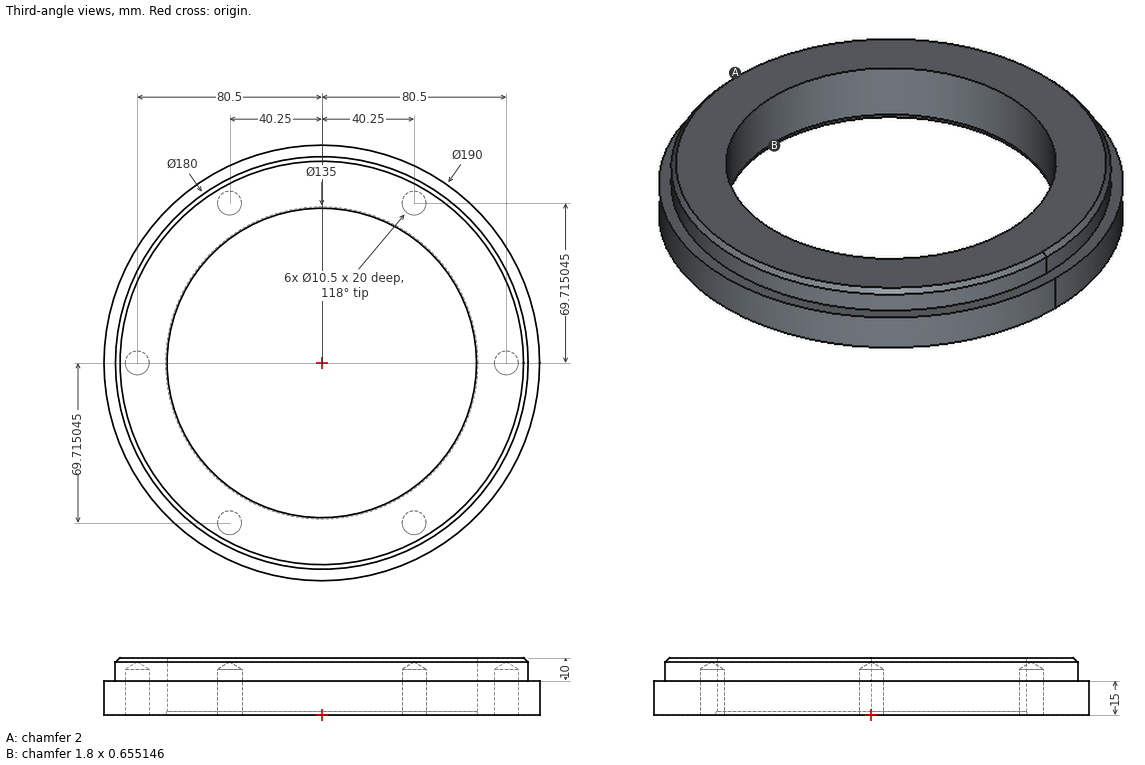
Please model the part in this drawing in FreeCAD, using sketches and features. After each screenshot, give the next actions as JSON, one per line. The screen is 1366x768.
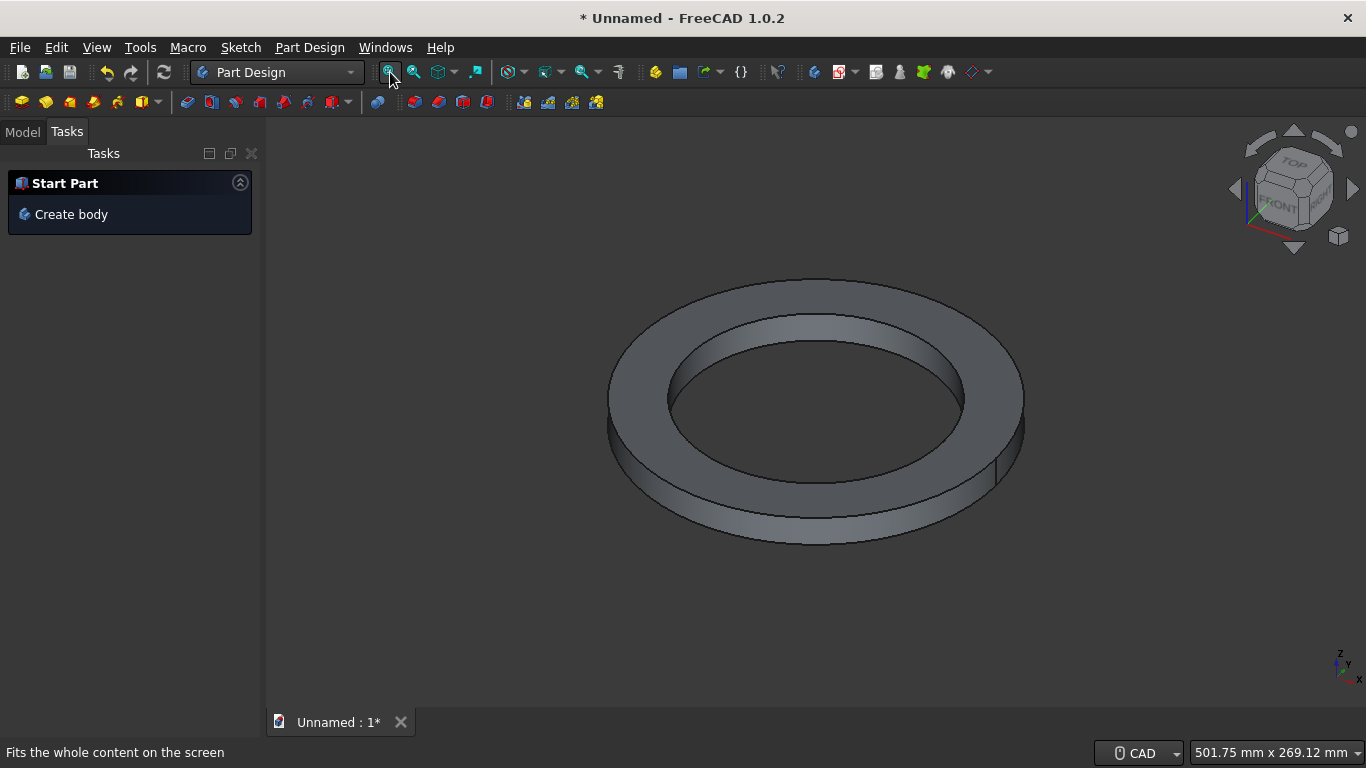
{"action": "left_click", "coordinate": [971, 449]}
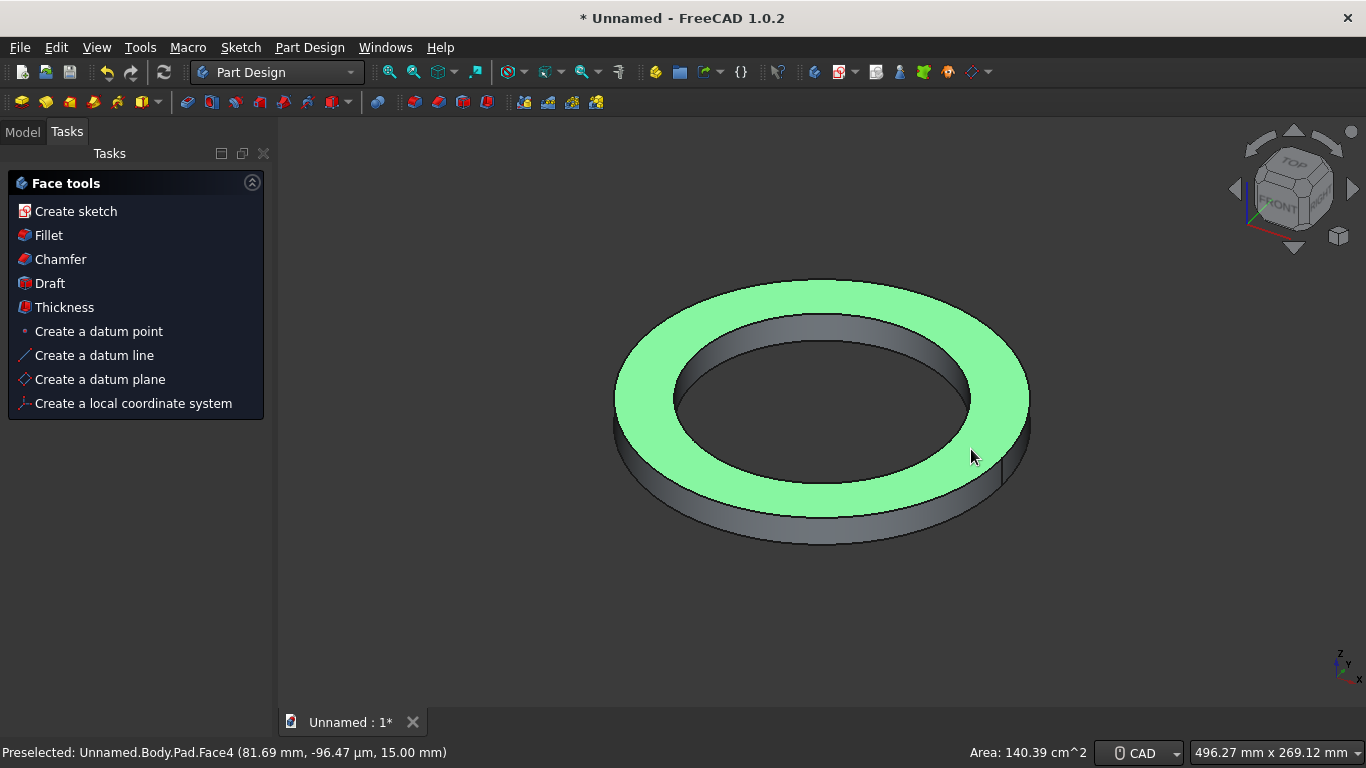
{"action": "left_click", "coordinate": [840, 72]}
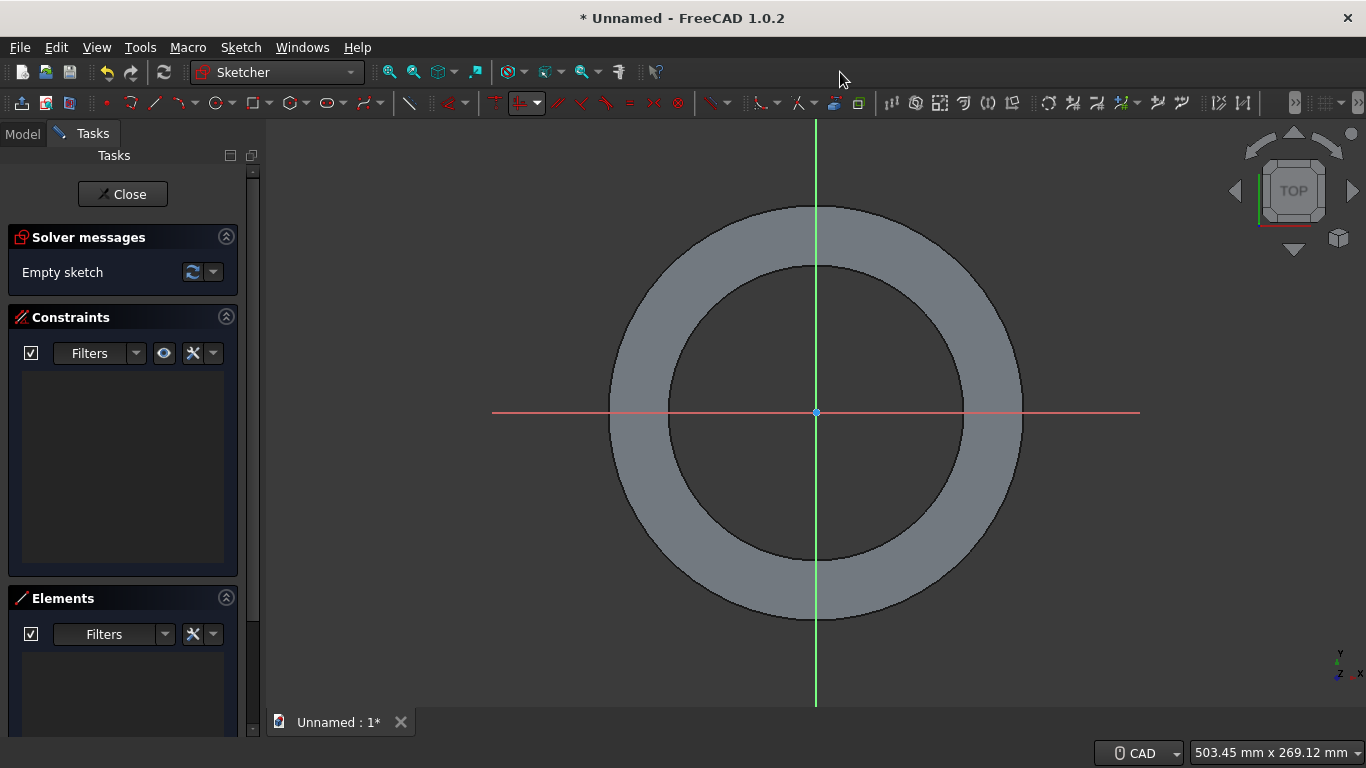
{"action": "left_click", "coordinate": [216, 104]}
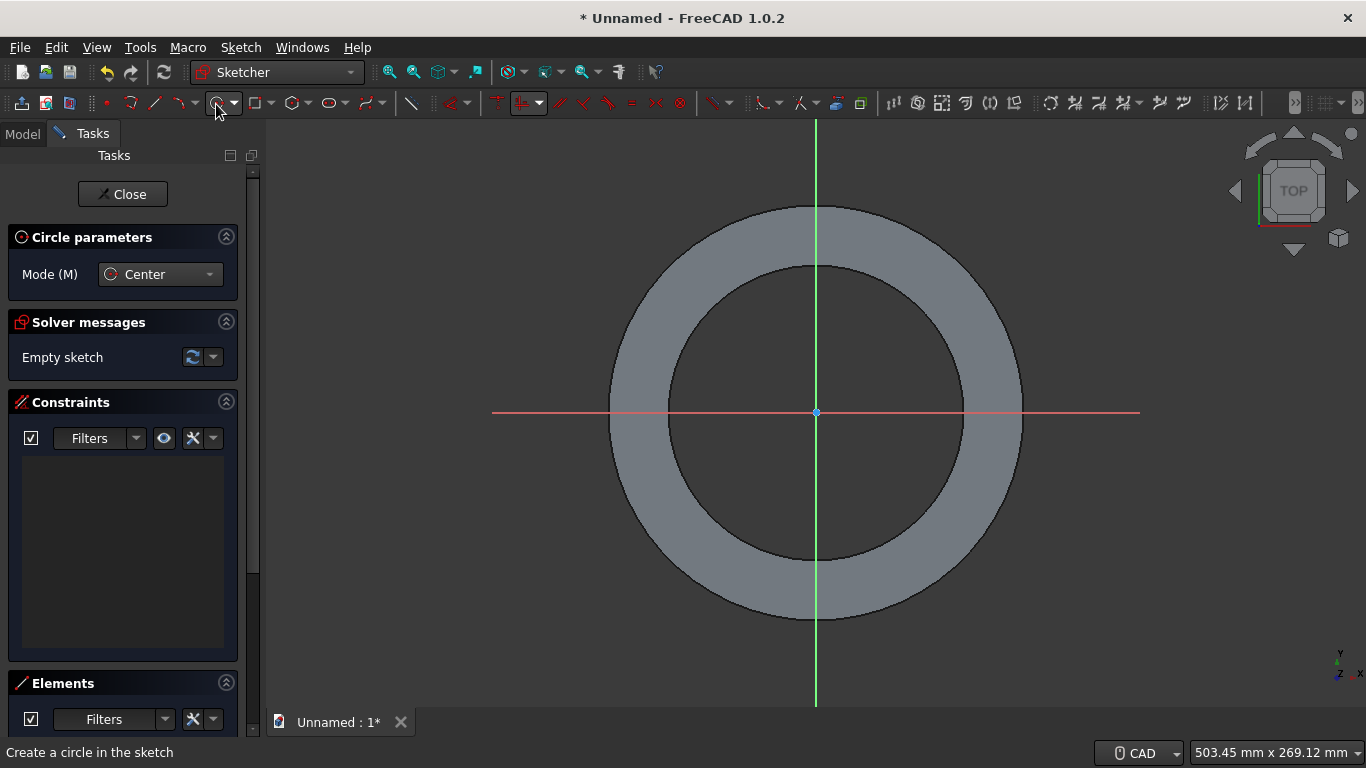
{"action": "left_click", "coordinate": [816, 413]}
{"action": "left_click", "coordinate": [955, 274]}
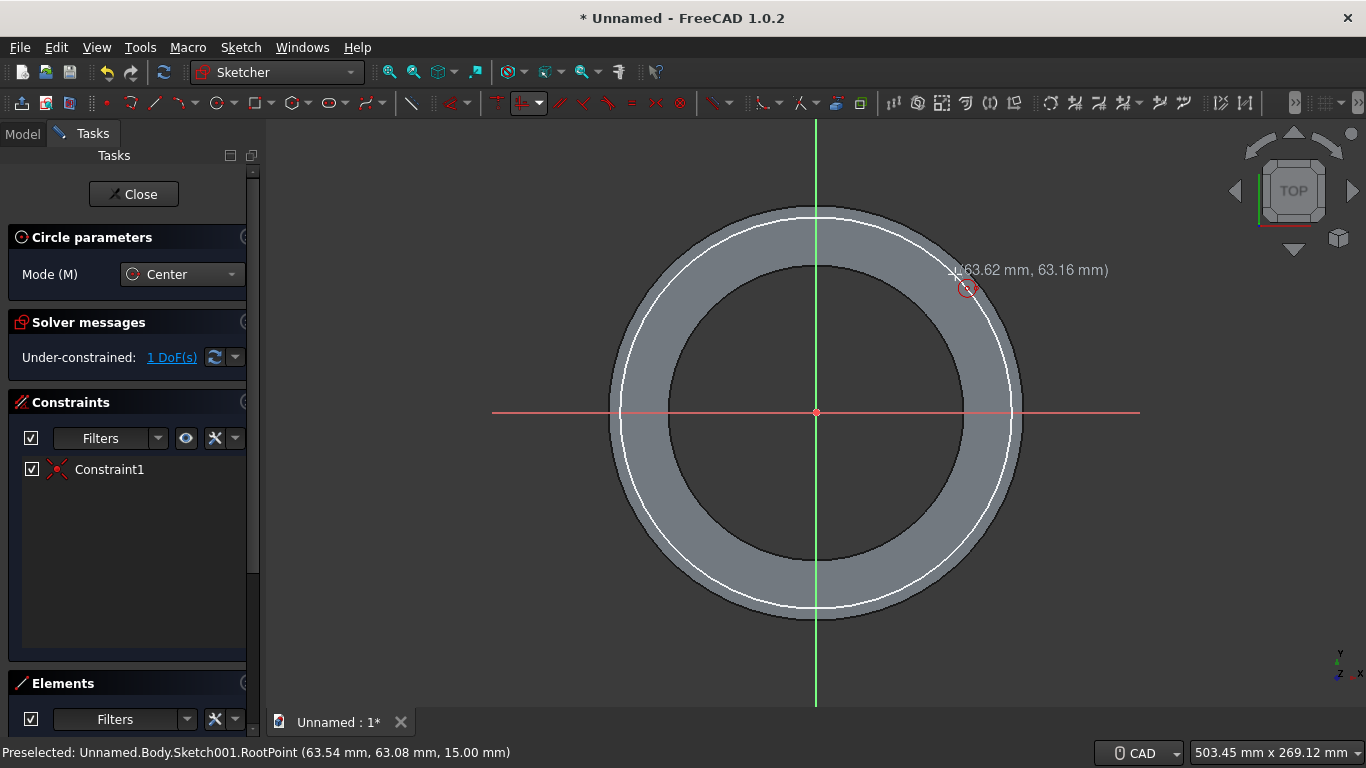
{"action": "left_click", "coordinate": [816, 413]}
{"action": "left_click", "coordinate": [920, 309]}
{"action": "key", "text": "Escape"}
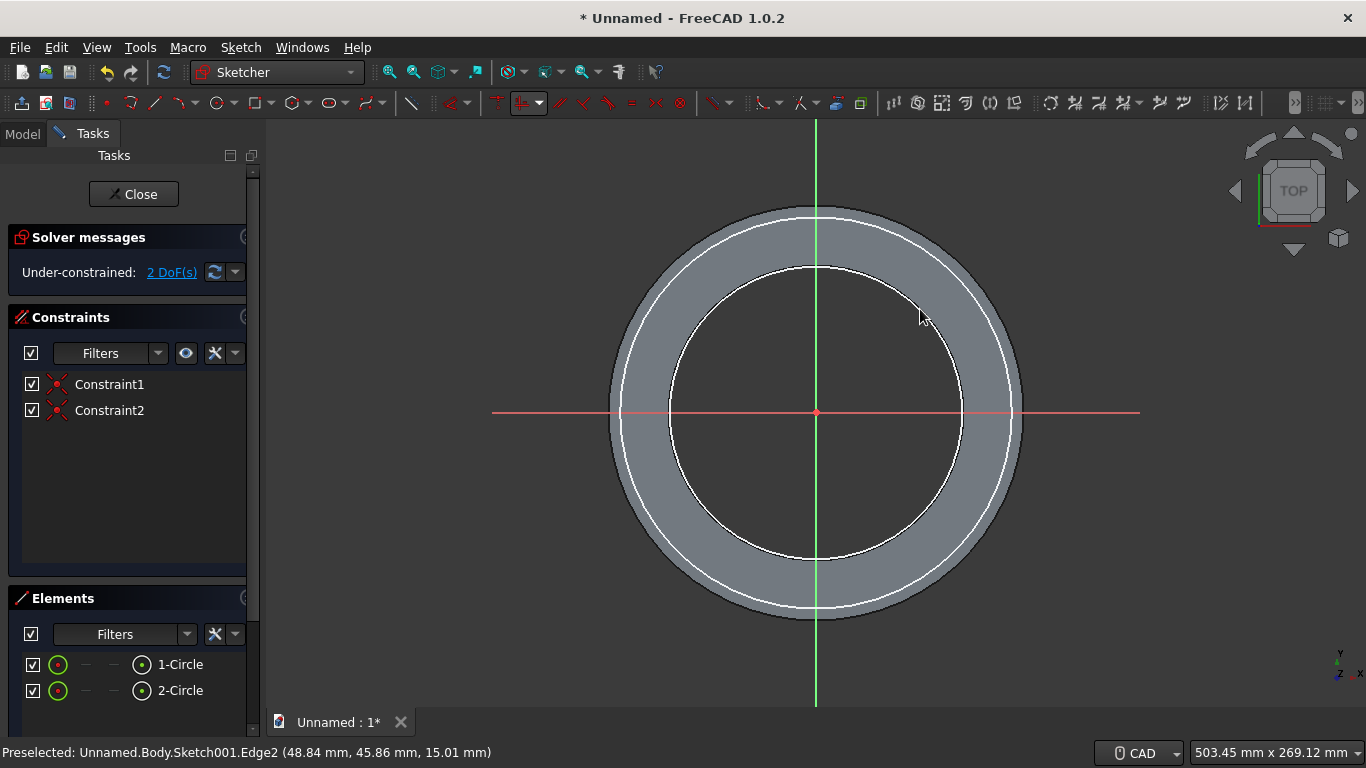
{"action": "left_click", "coordinate": [450, 104]}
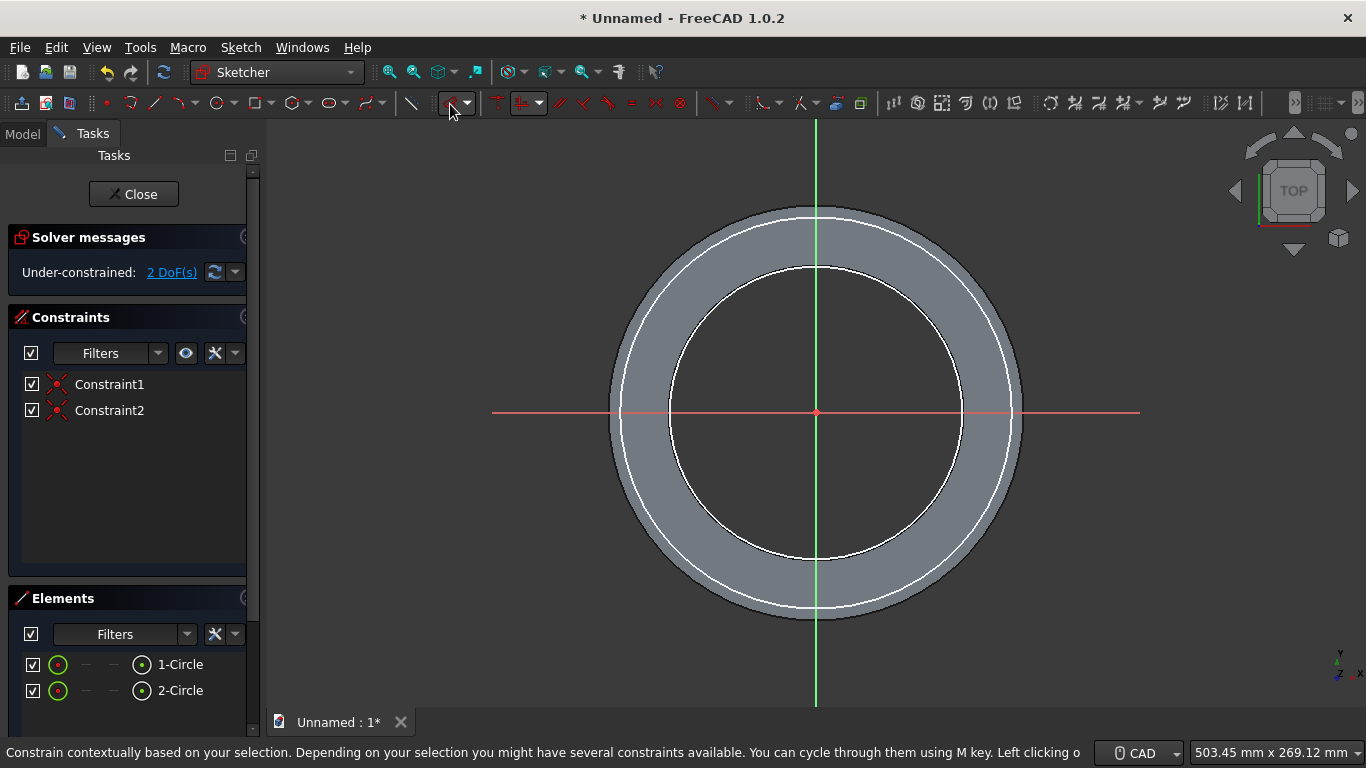
{"action": "left_click", "coordinate": [954, 274]}
{"action": "left_click", "coordinate": [977, 251]}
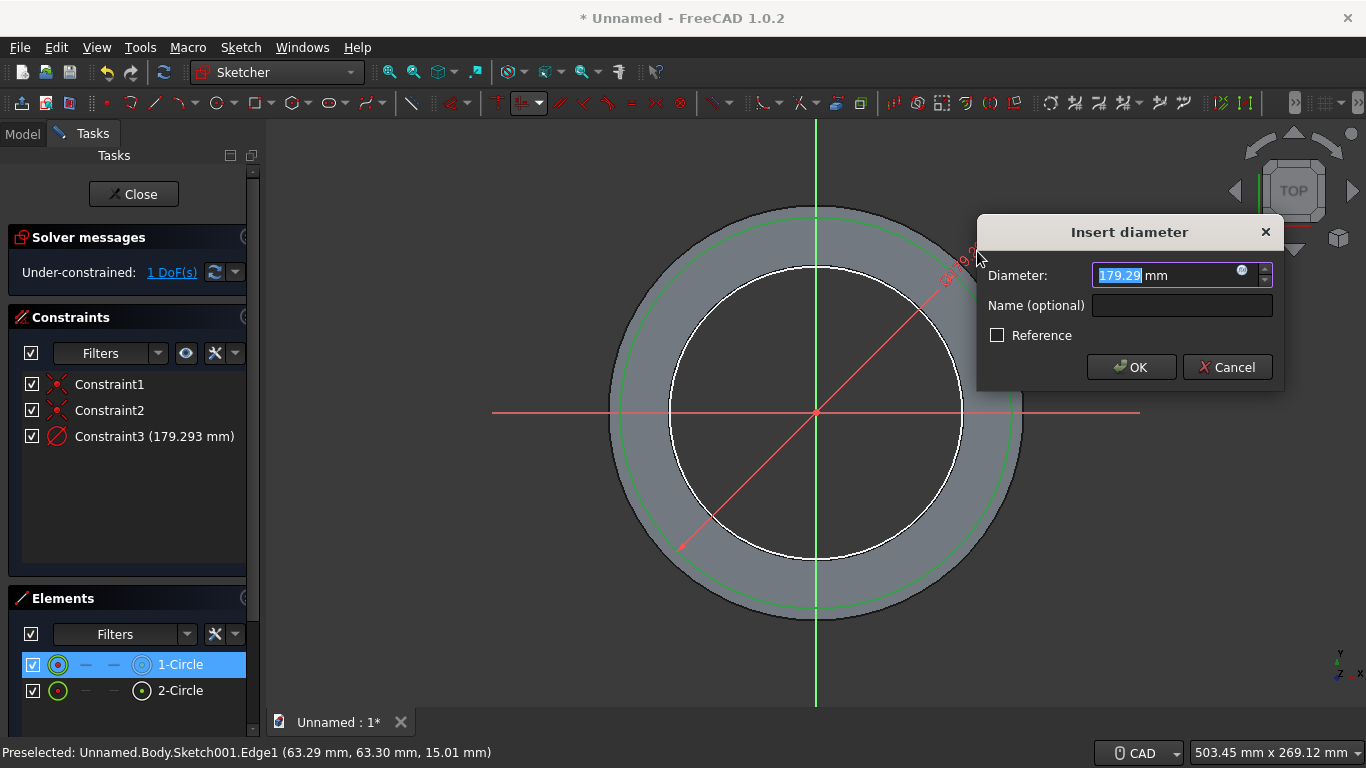
{"action": "type", "text": "180"}
{"action": "key", "text": "Return"}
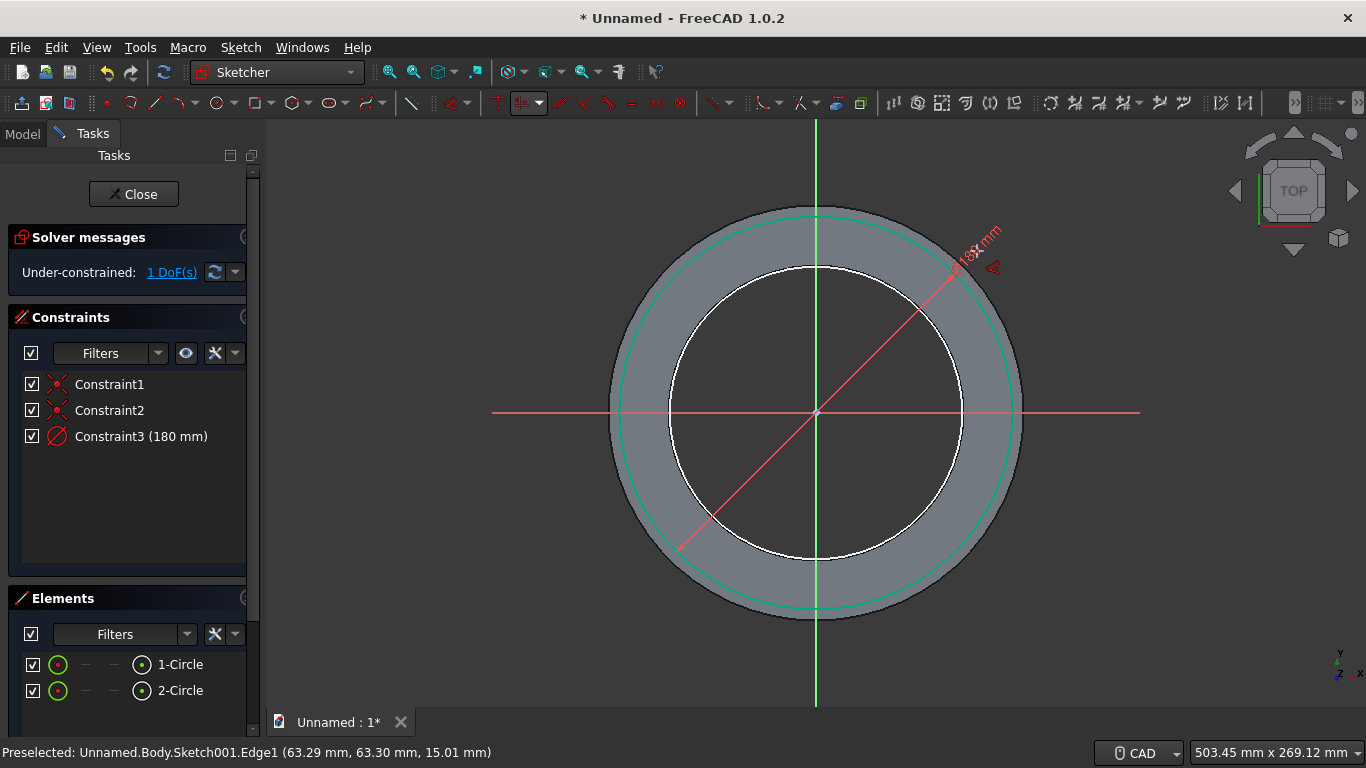
{"action": "left_click", "coordinate": [919, 309]}
{"action": "left_click", "coordinate": [942, 286]}